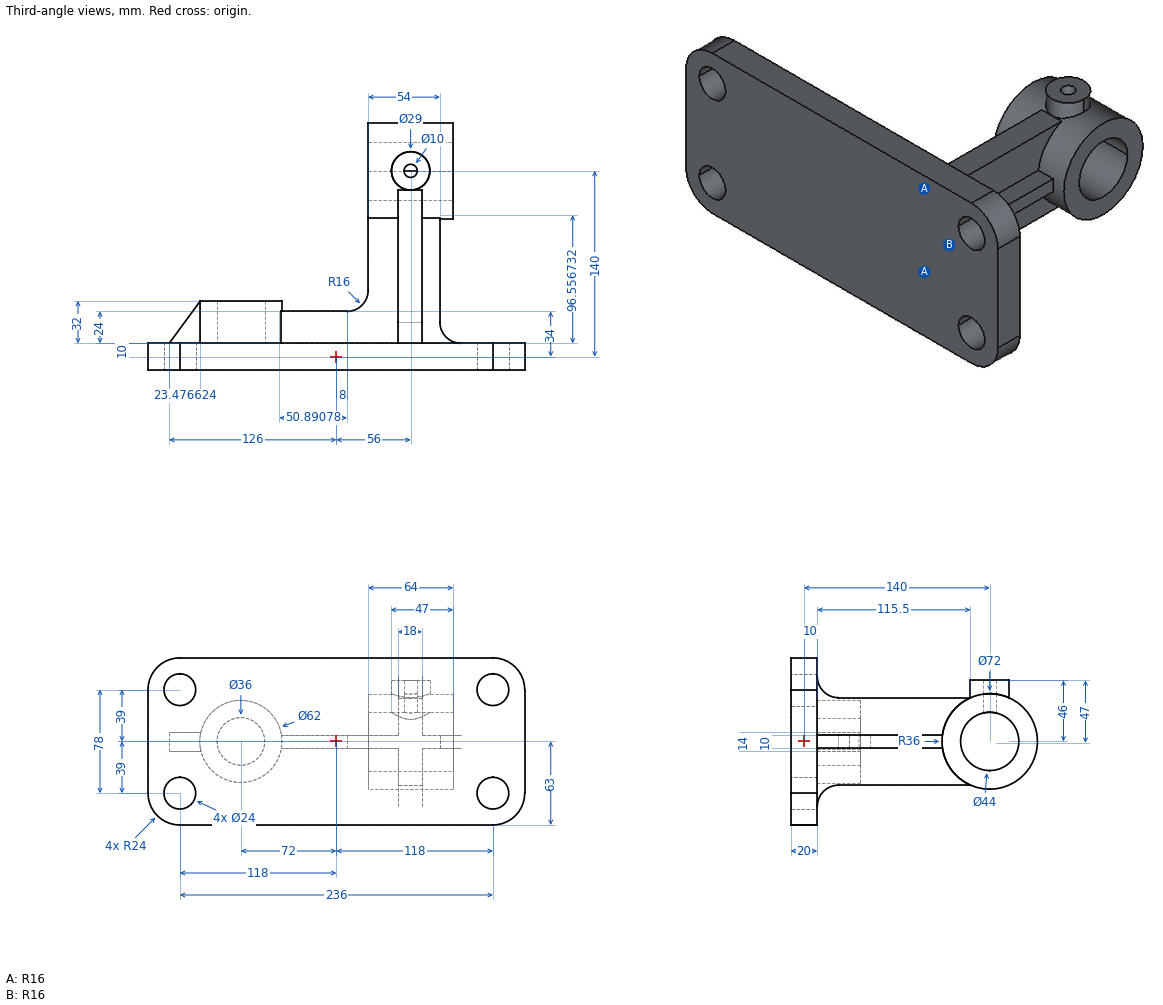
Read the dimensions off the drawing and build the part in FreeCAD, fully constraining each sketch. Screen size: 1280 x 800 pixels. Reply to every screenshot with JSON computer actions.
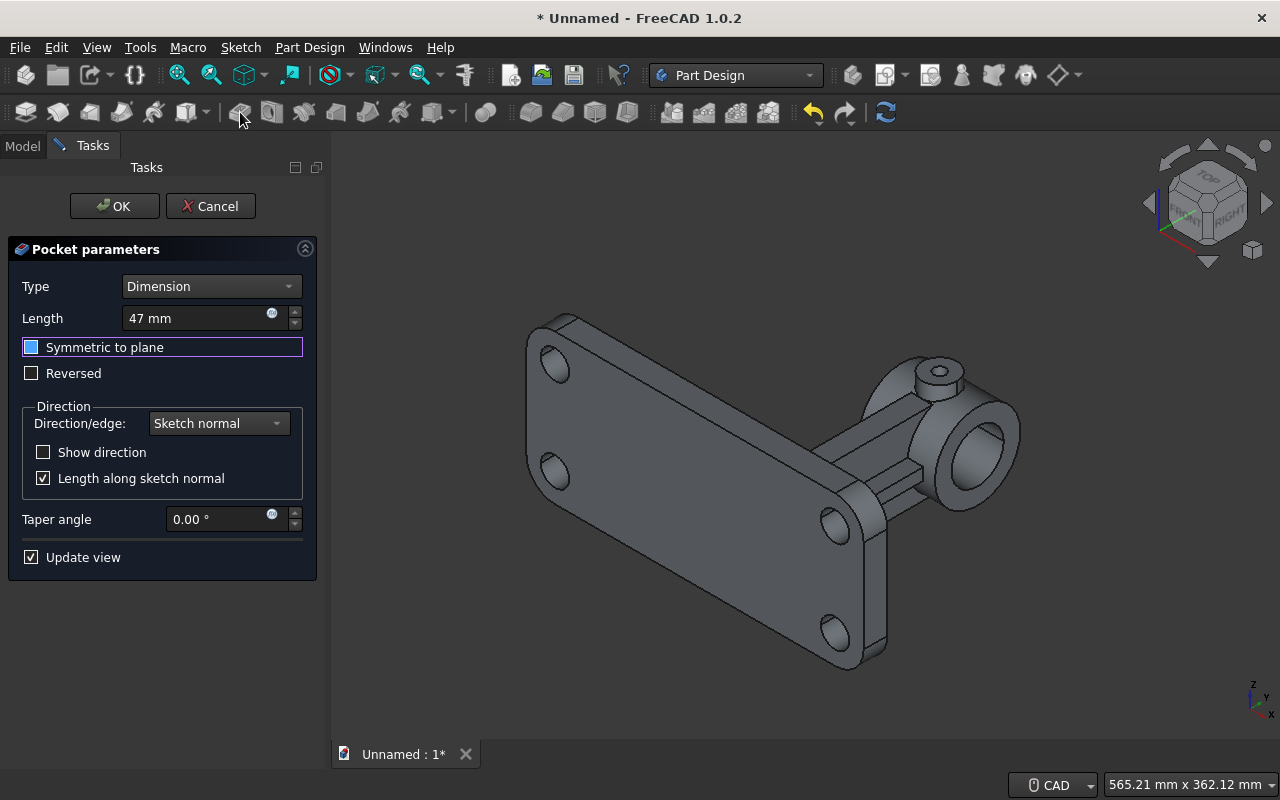
{"action": "left_click", "coordinate": [115, 206]}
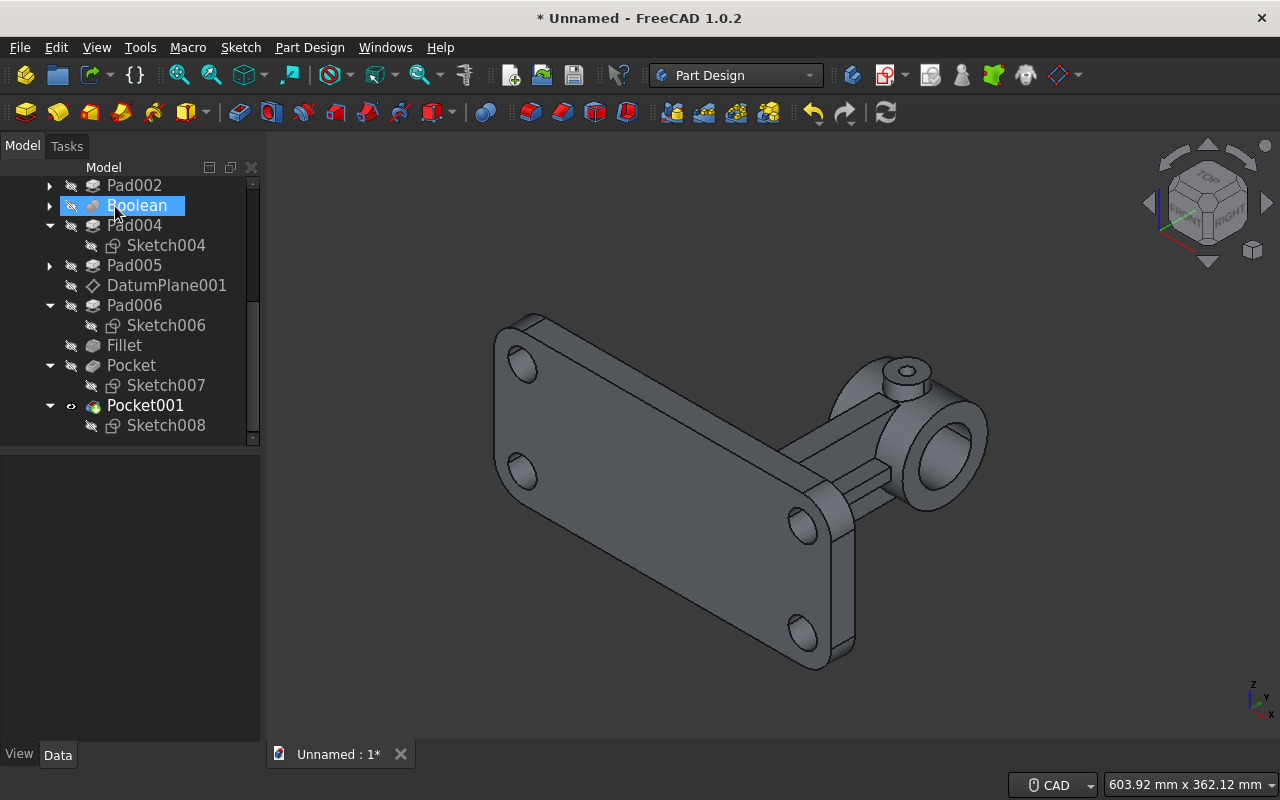
{"action": "scroll", "coordinate": [140, 301], "scroll_direction": "down", "scroll_amount": 3}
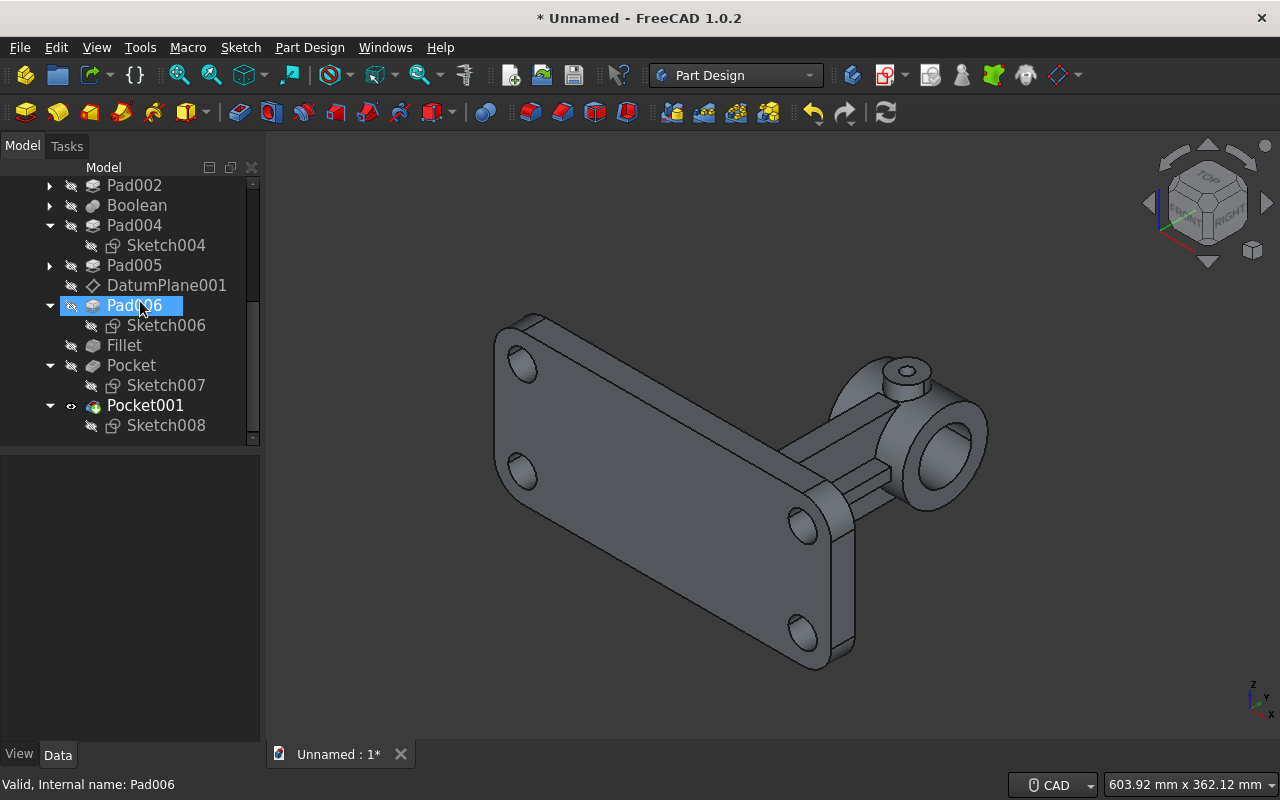
{"action": "scroll", "coordinate": [140, 301], "scroll_direction": "up", "scroll_amount": 15}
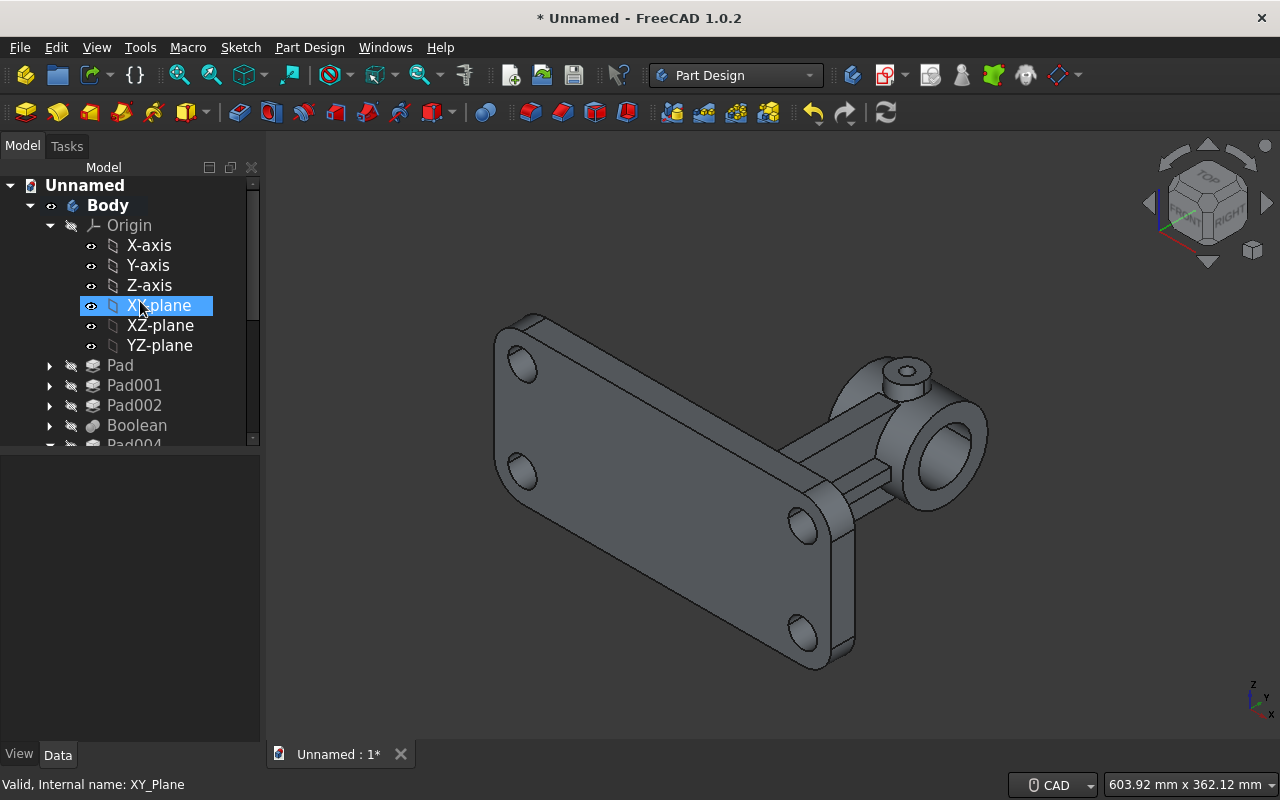
{"action": "left_click", "coordinate": [136, 306]}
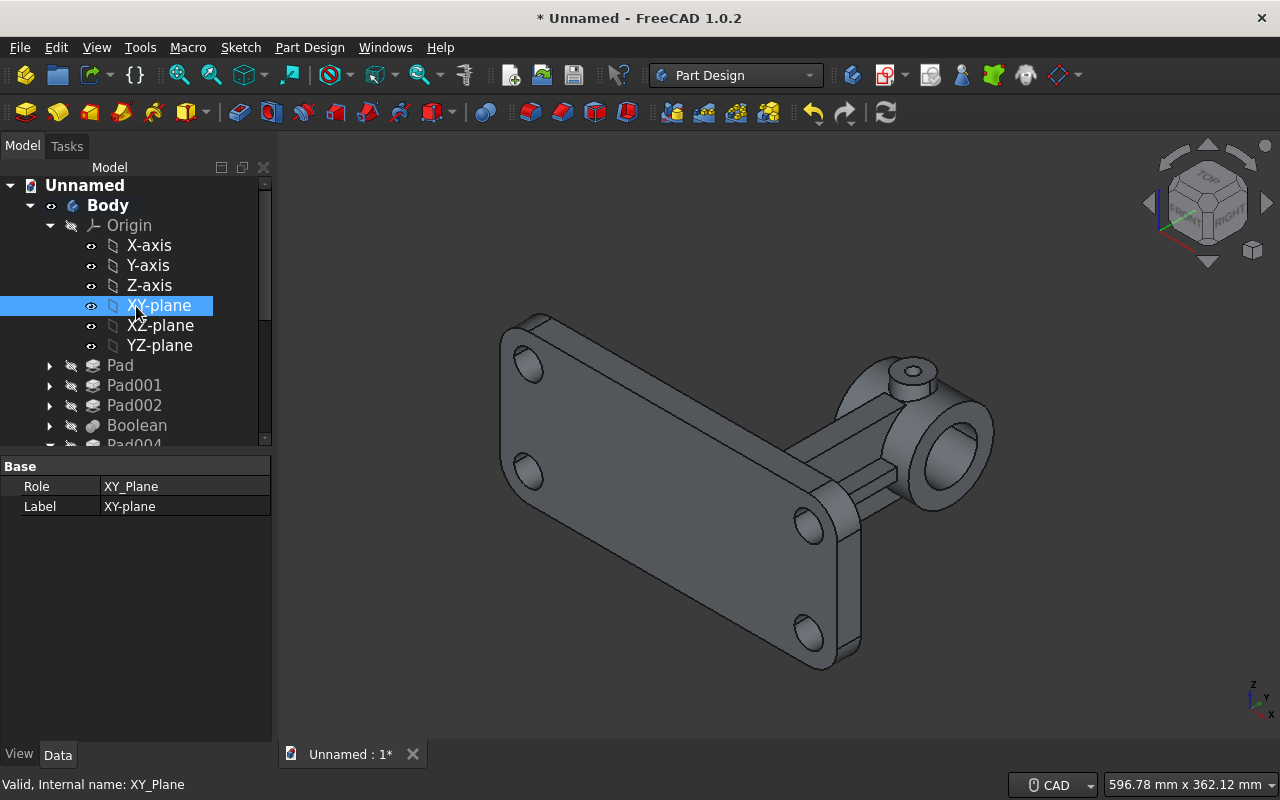
{"action": "left_click", "coordinate": [1058, 76]}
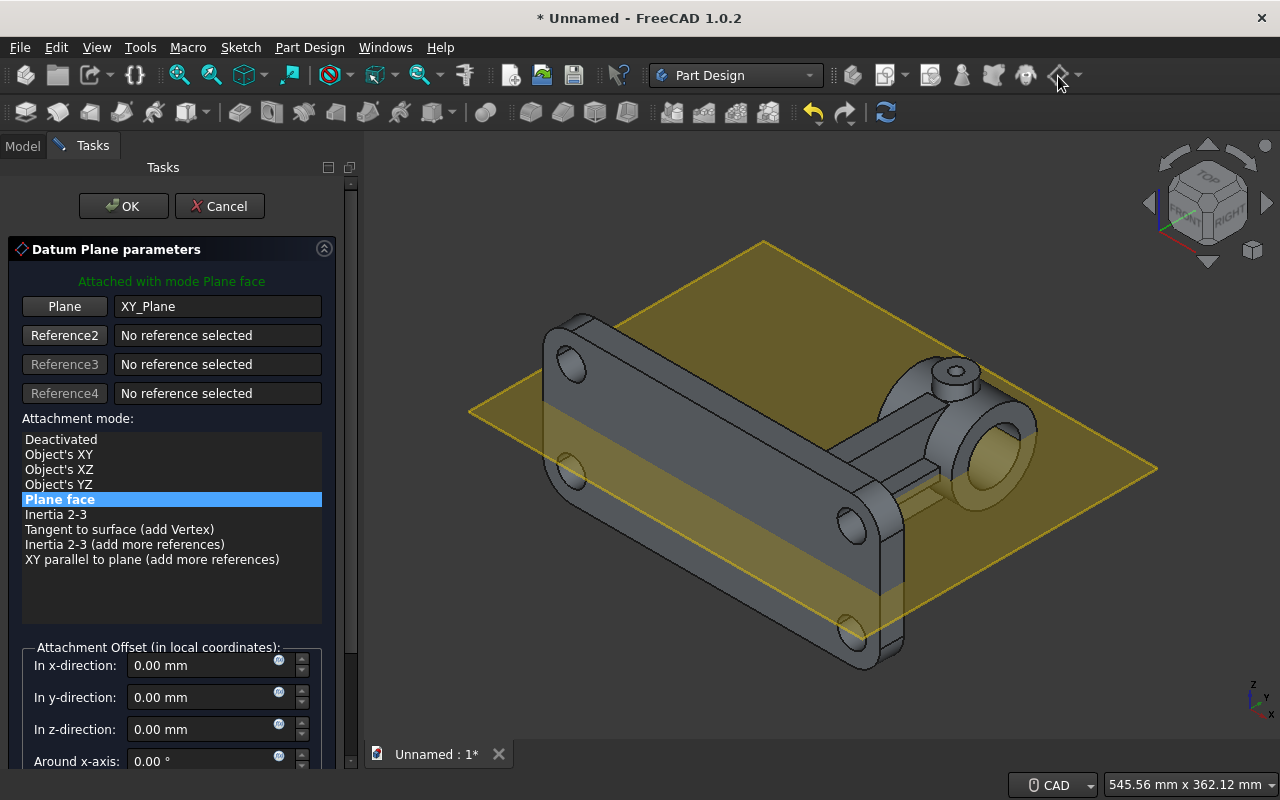
{"action": "triple_click", "coordinate": [210, 729]}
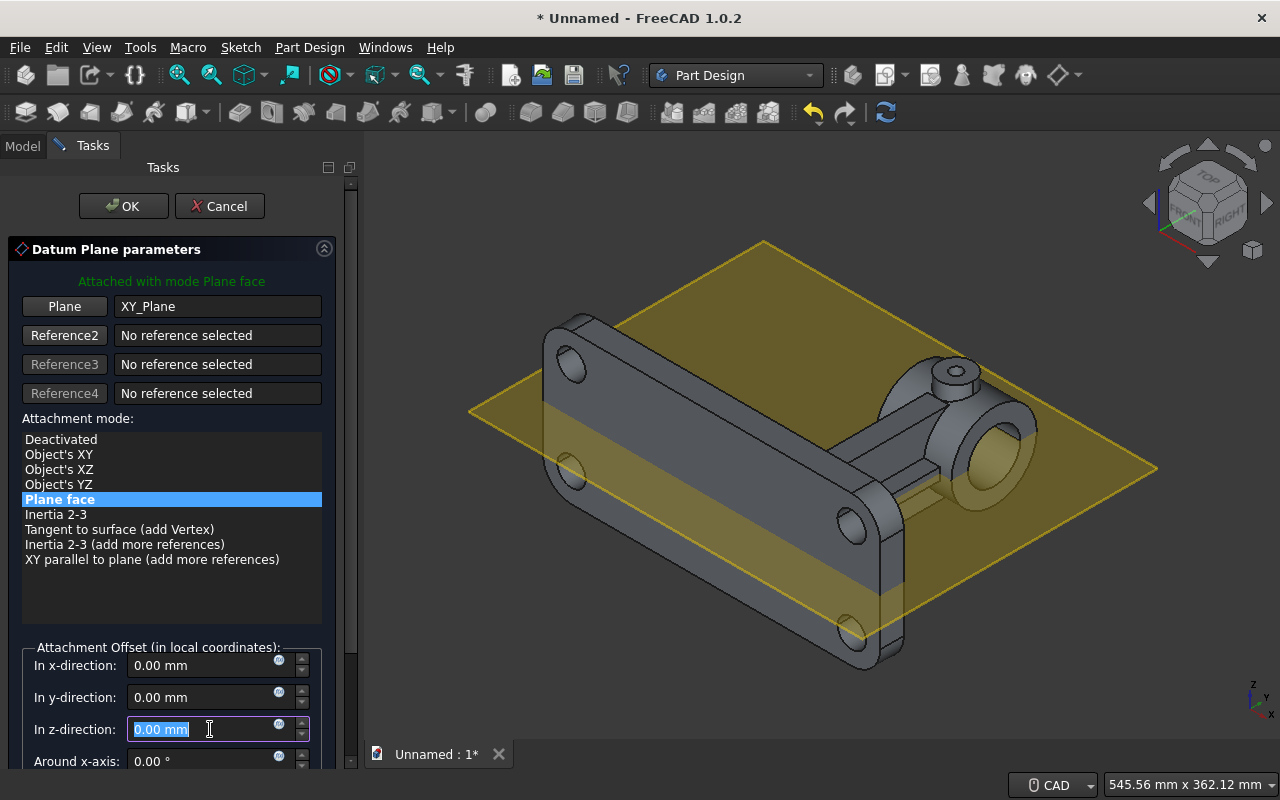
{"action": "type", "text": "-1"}
{"action": "key", "text": "Tab"}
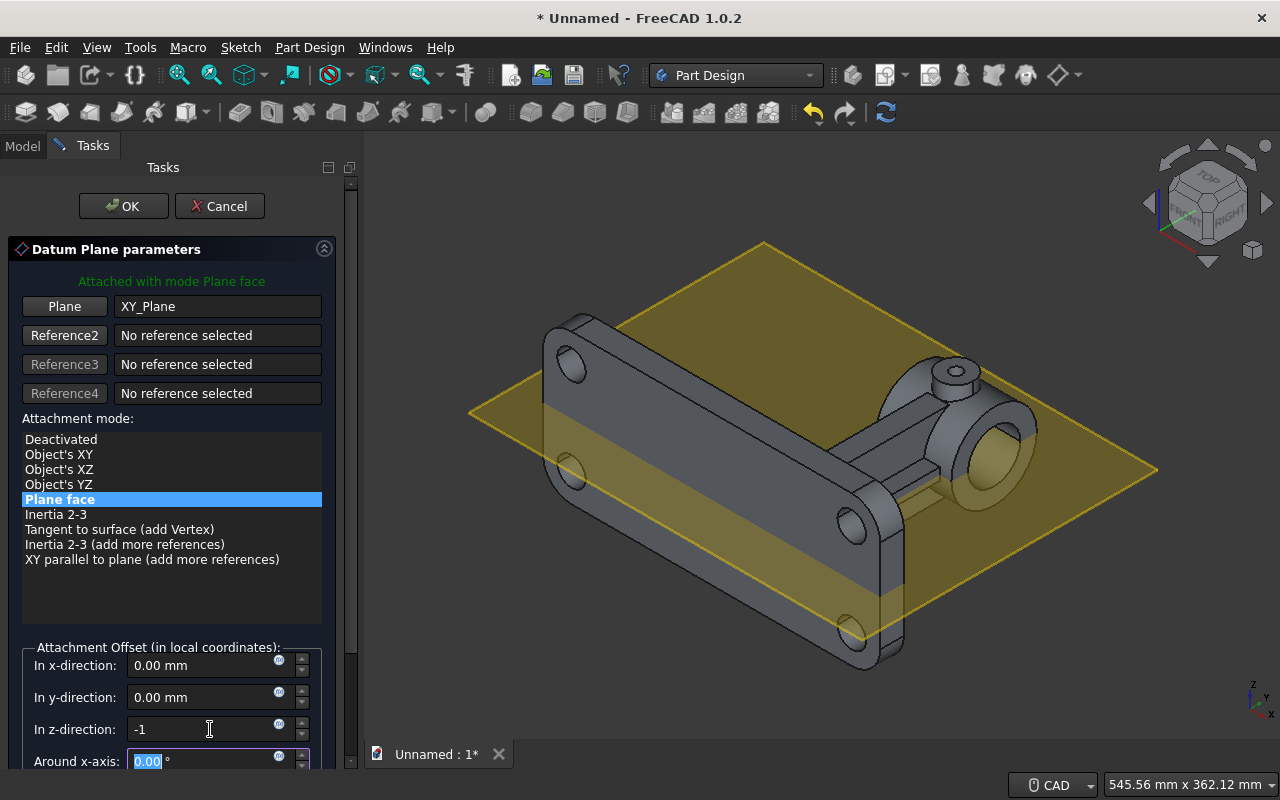
{"action": "left_click", "coordinate": [124, 206]}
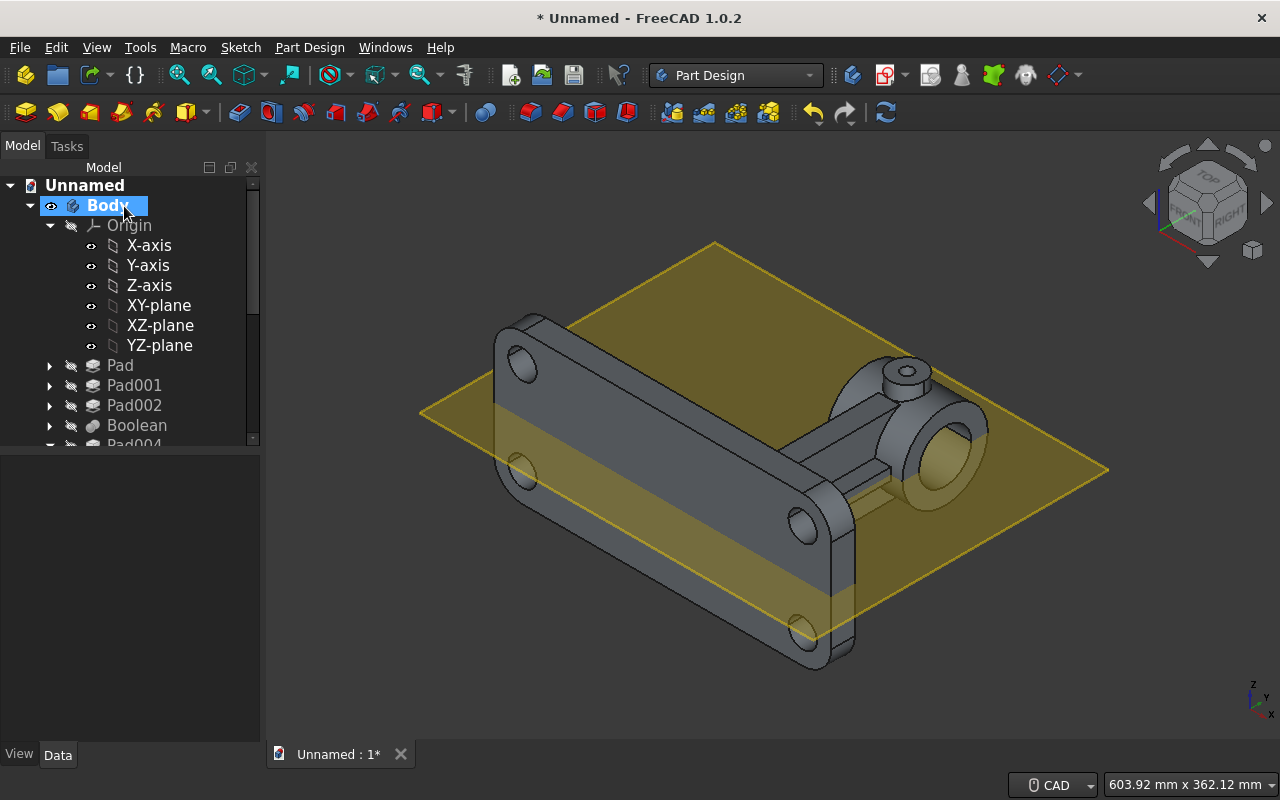
{"action": "scroll", "coordinate": [100, 321], "scroll_direction": "down", "scroll_amount": 3}